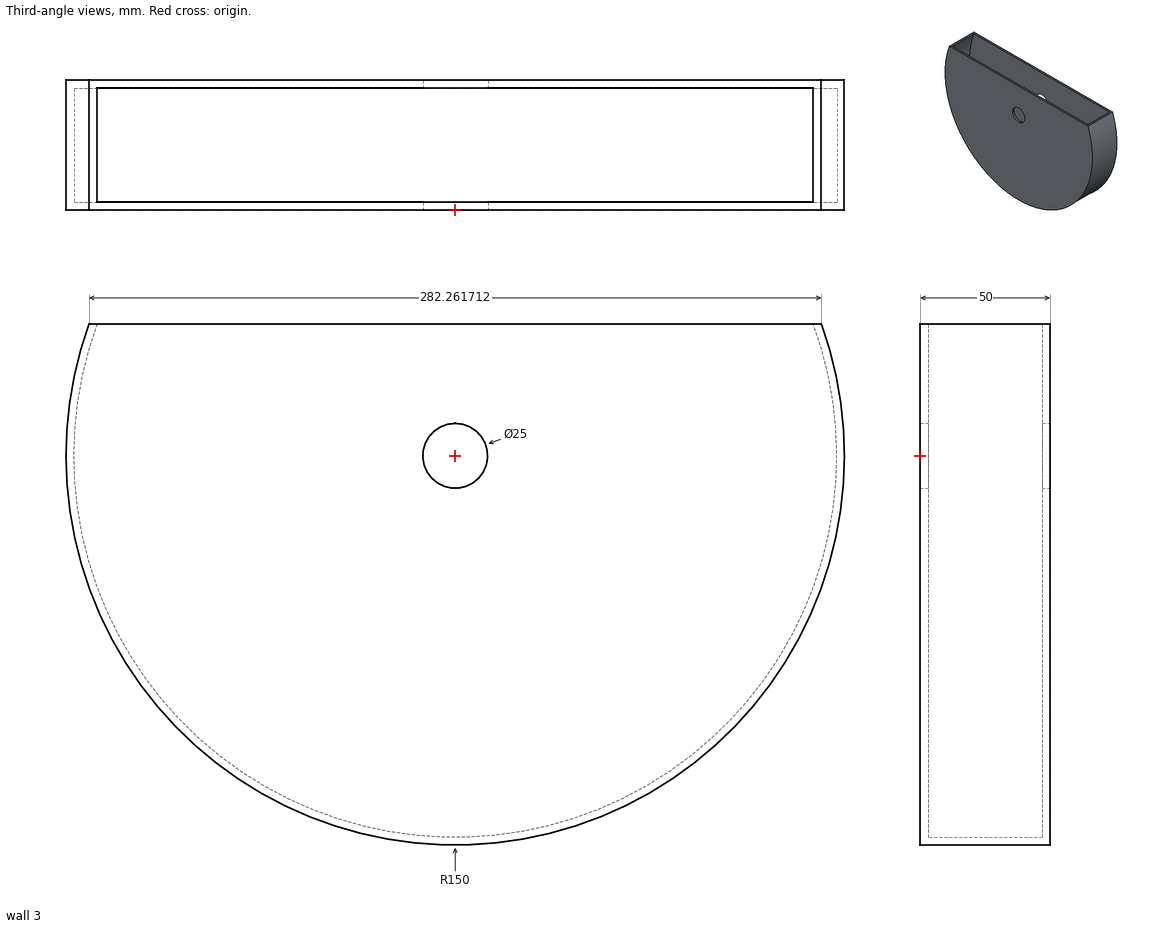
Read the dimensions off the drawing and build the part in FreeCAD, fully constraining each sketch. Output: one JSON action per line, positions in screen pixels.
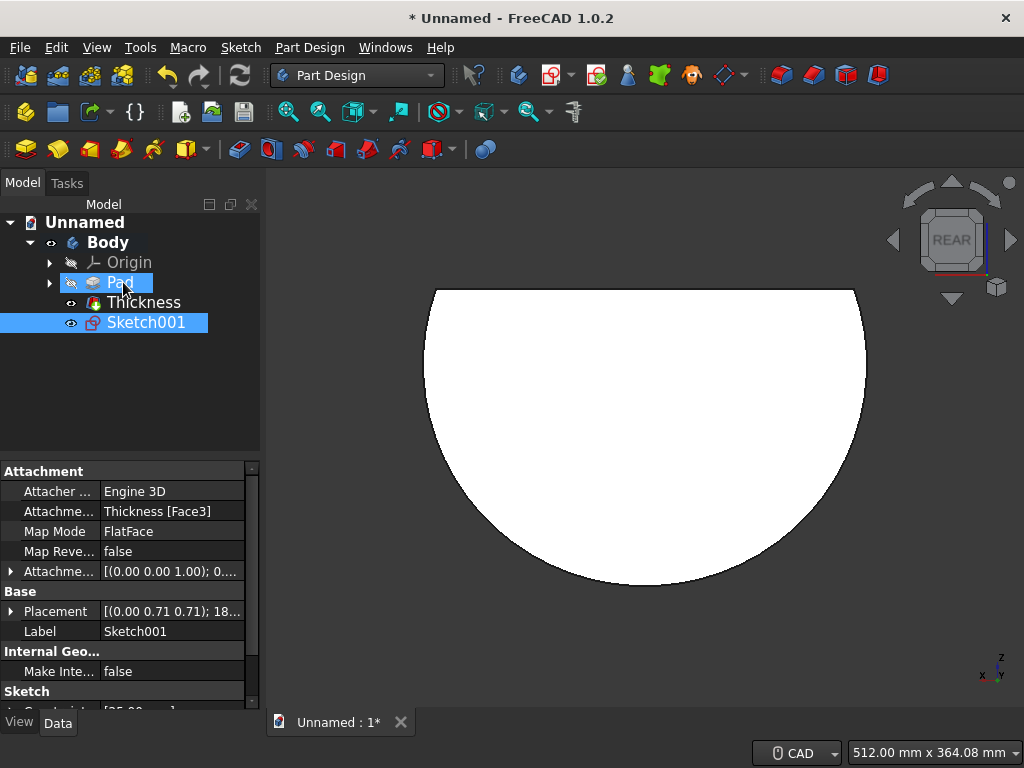
{"action": "left_click", "coordinate": [240, 150]}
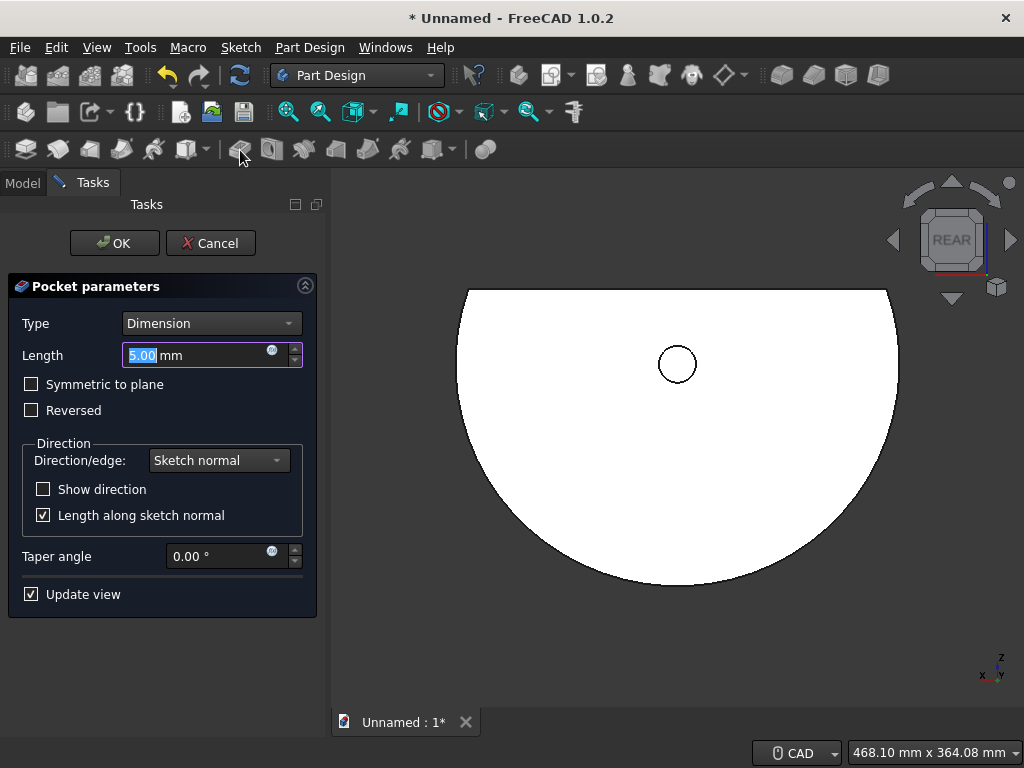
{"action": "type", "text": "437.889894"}
{"action": "key", "text": "Tab"}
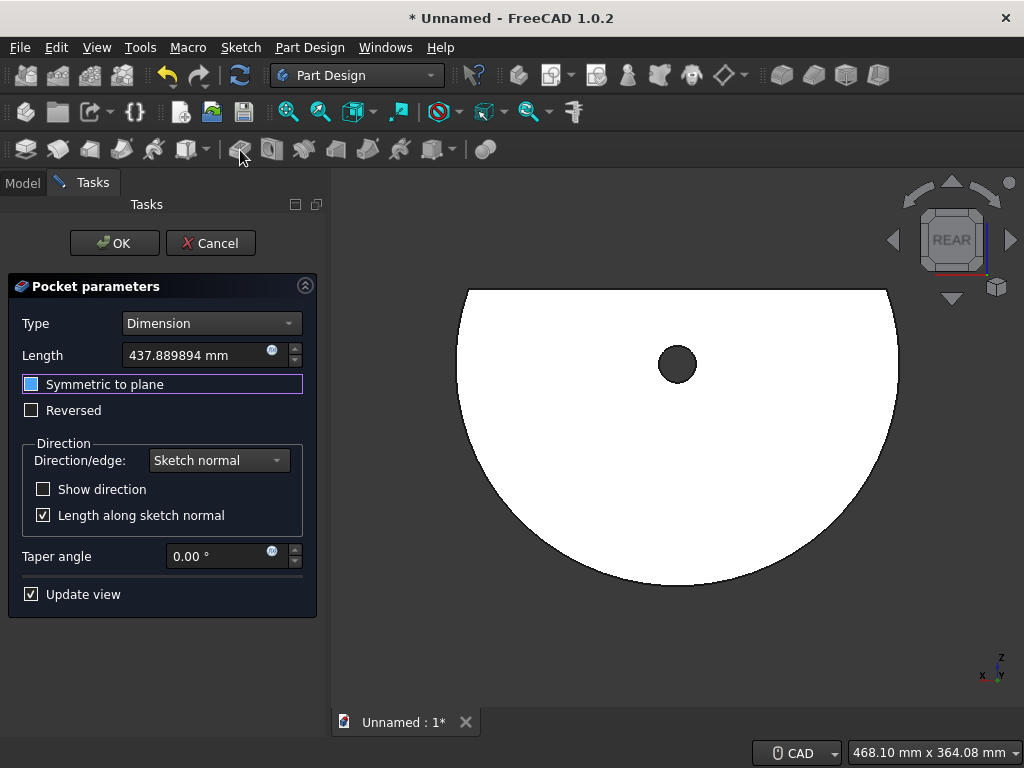
{"action": "left_click", "coordinate": [30, 384]}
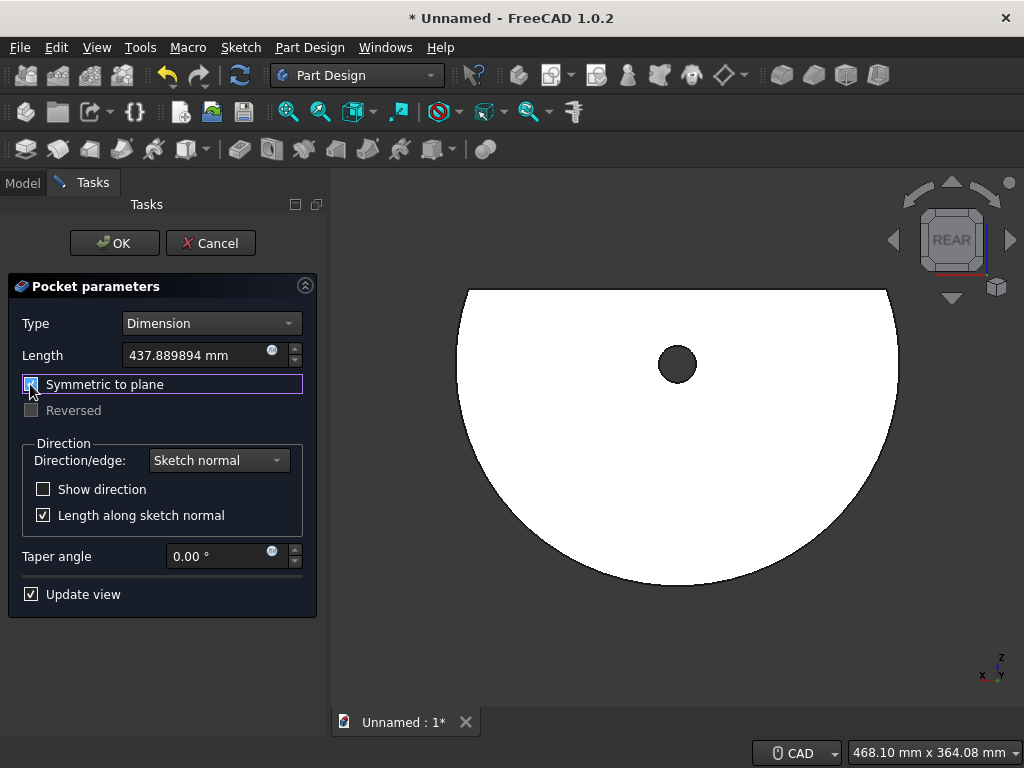
{"action": "left_click", "coordinate": [115, 243]}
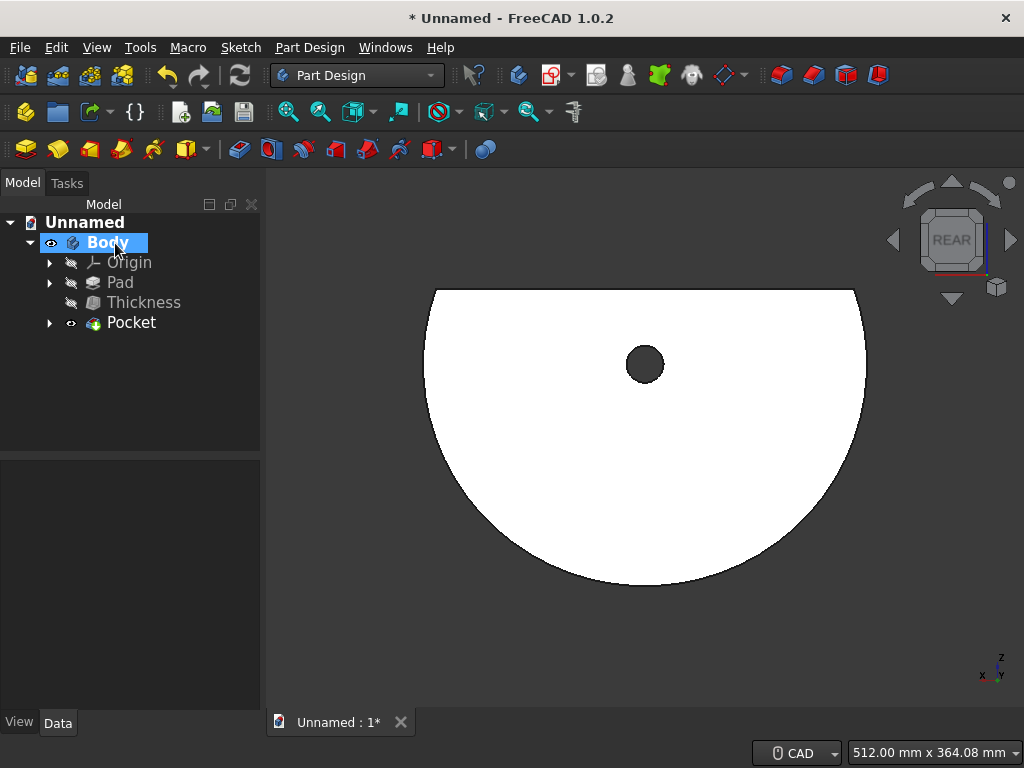
{"action": "key", "text": "0"}